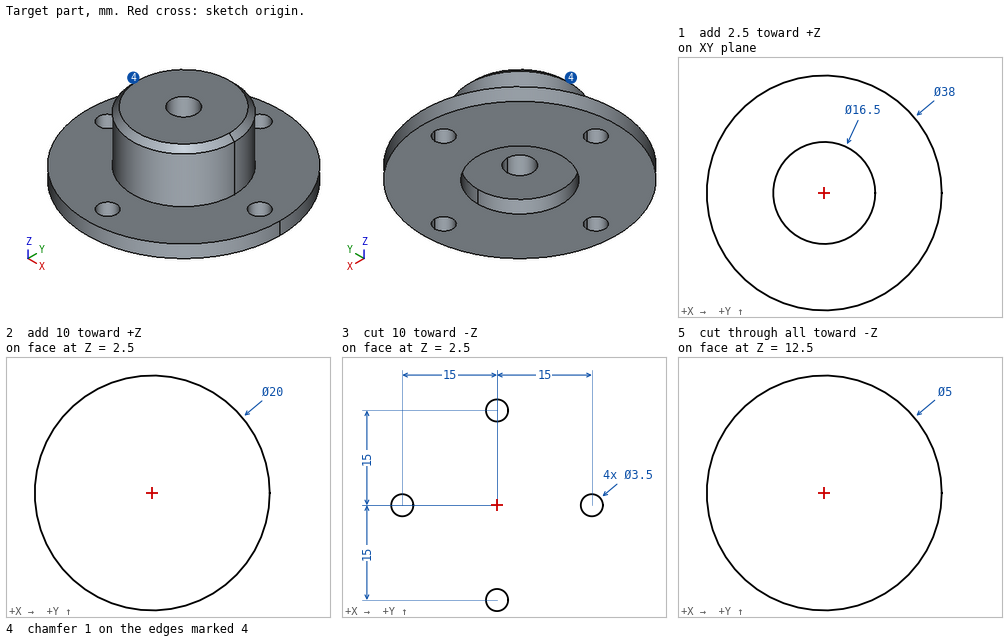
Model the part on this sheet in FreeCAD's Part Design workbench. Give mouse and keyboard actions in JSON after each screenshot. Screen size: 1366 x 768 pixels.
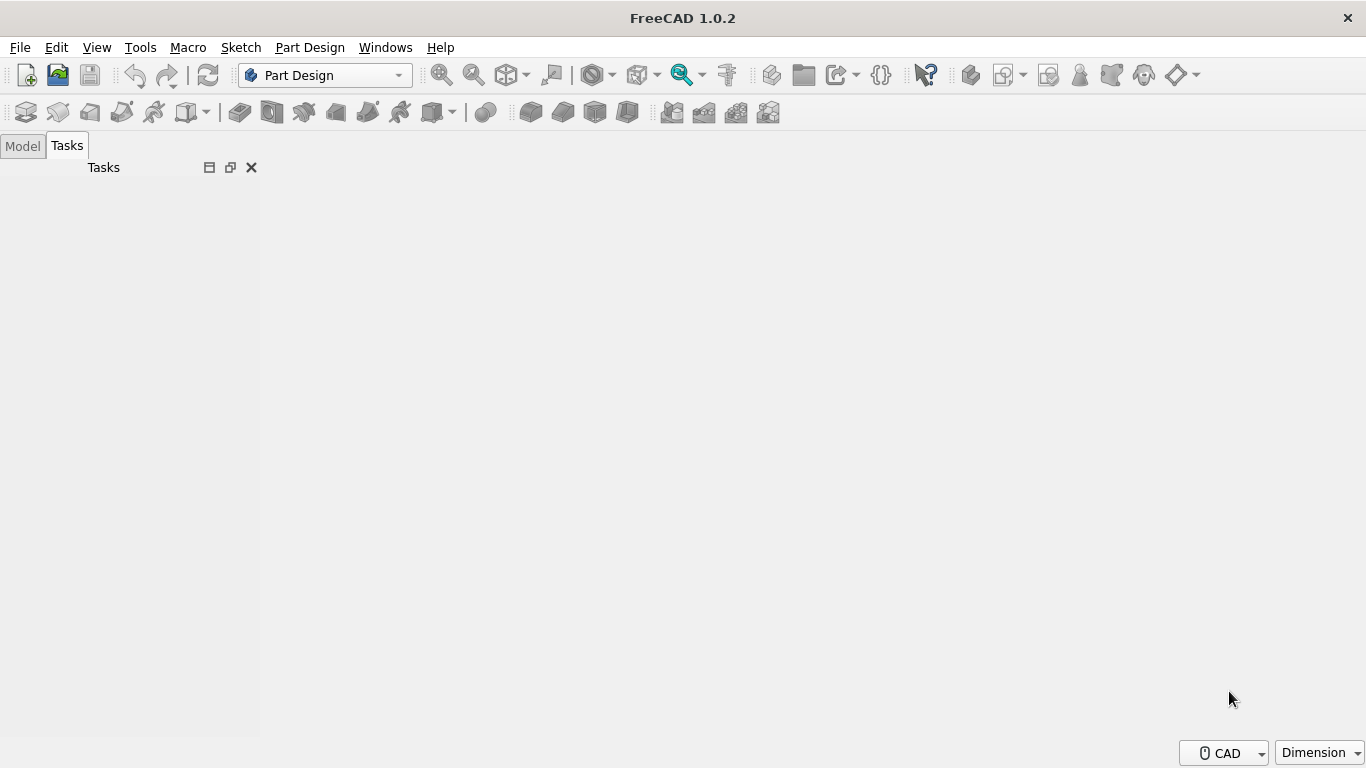
{"action": "key", "text": "ctrl+n"}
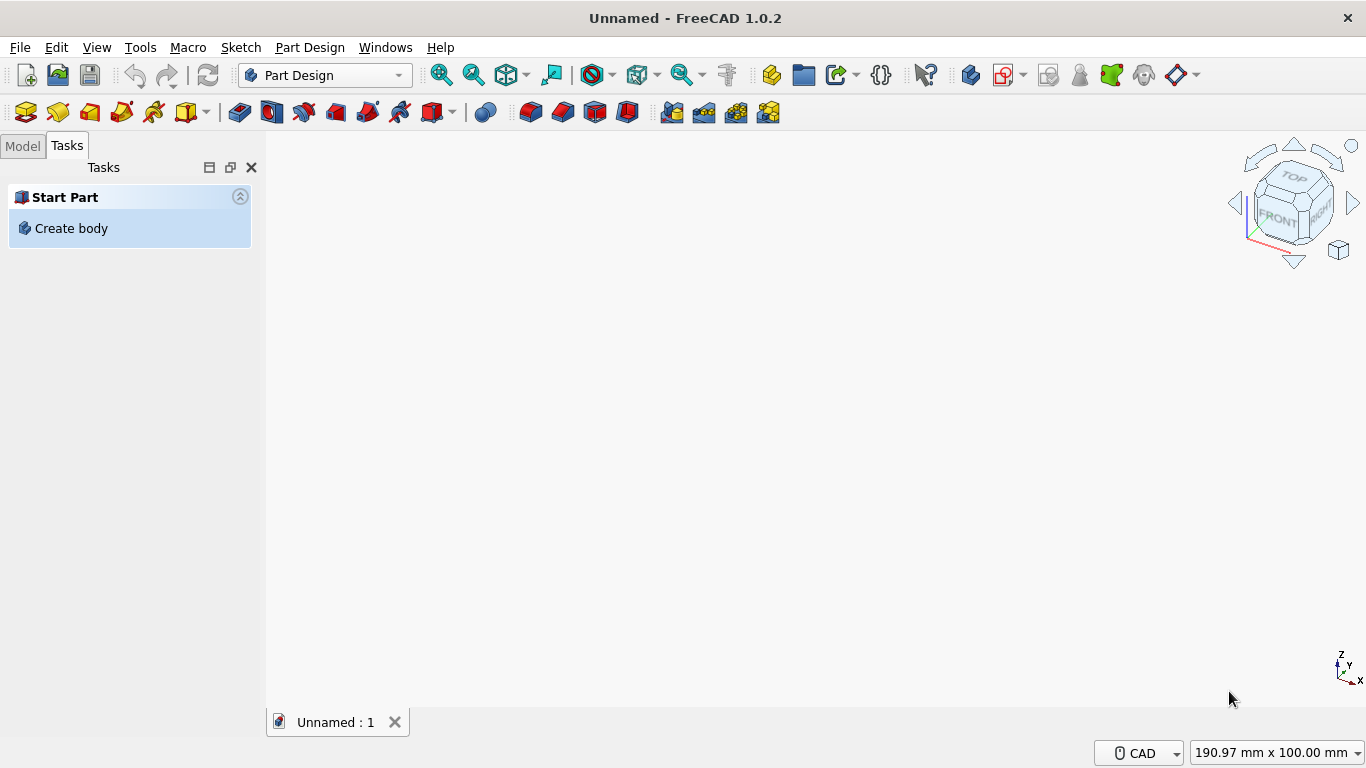
{"action": "left_click", "coordinate": [1004, 76]}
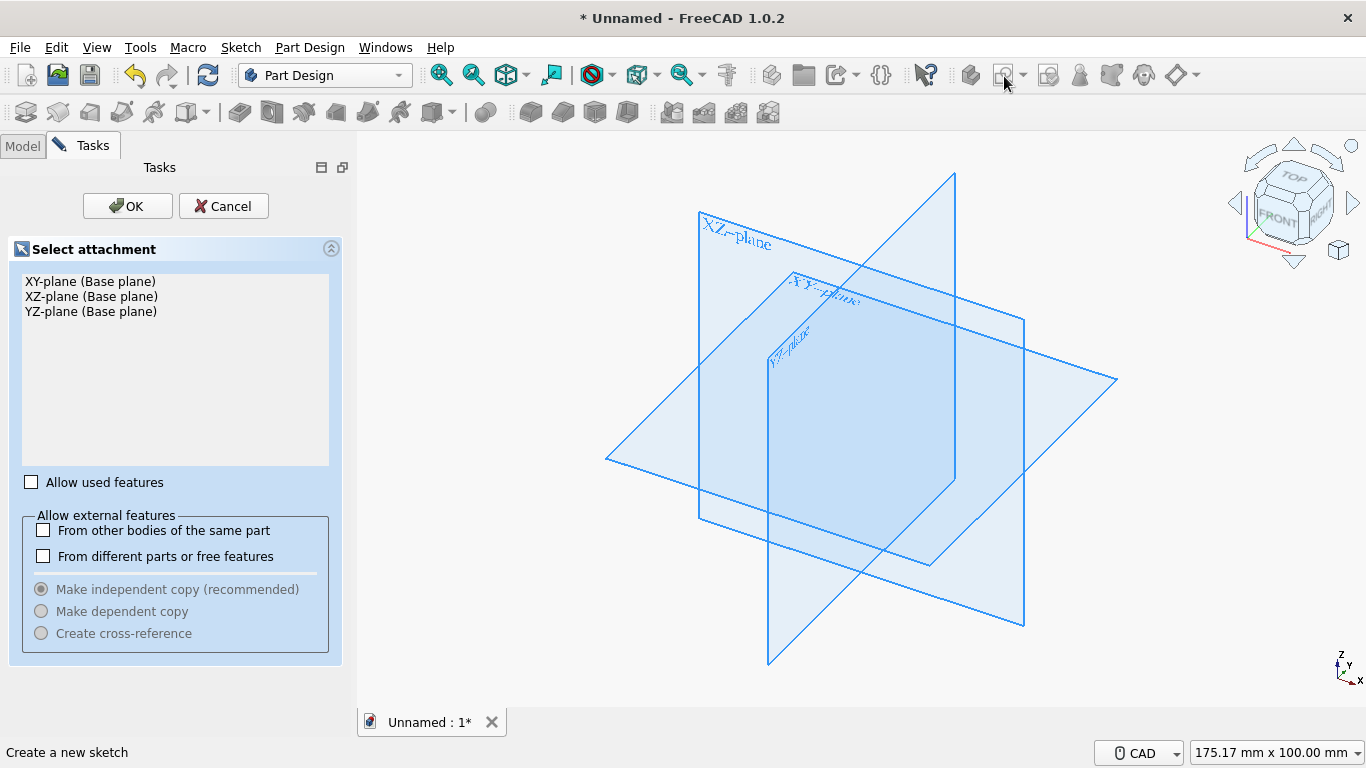
{"action": "left_click", "coordinate": [82, 282]}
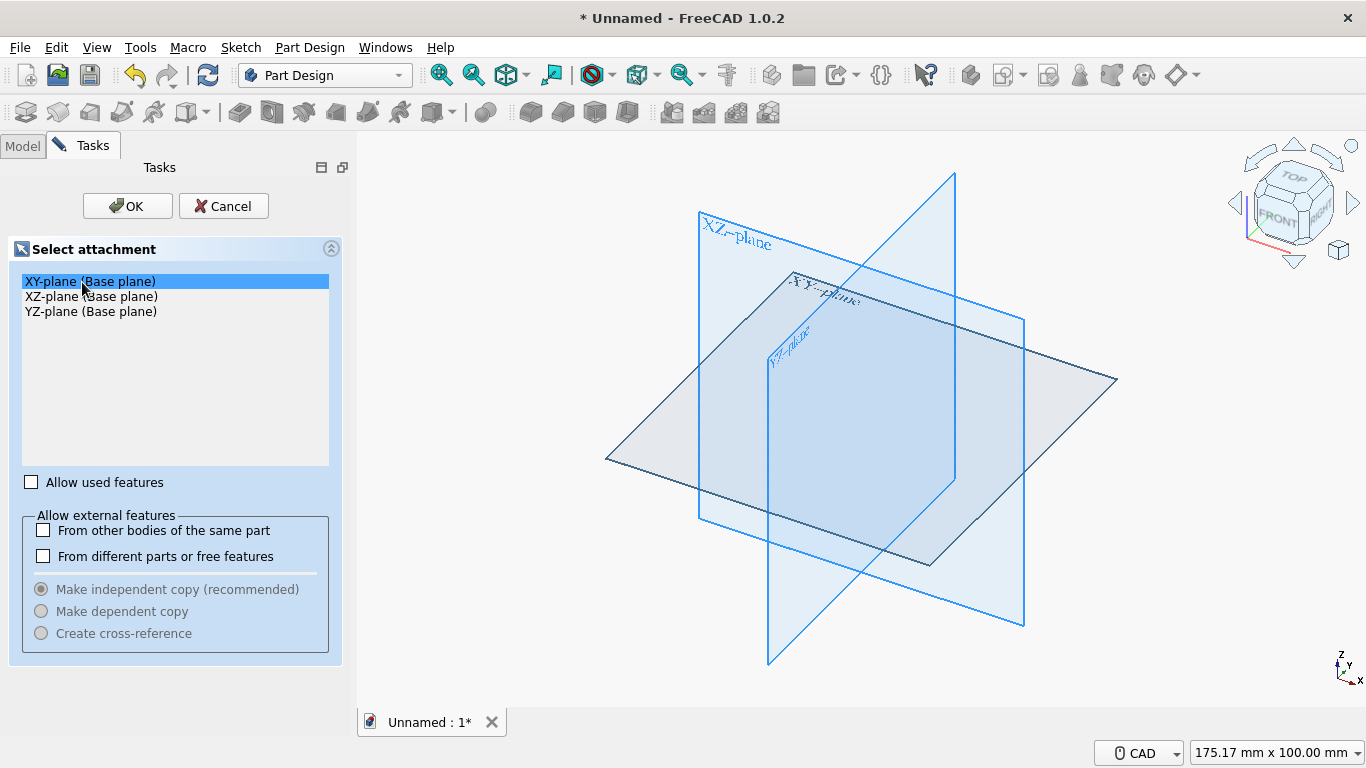
{"action": "left_click", "coordinate": [128, 206]}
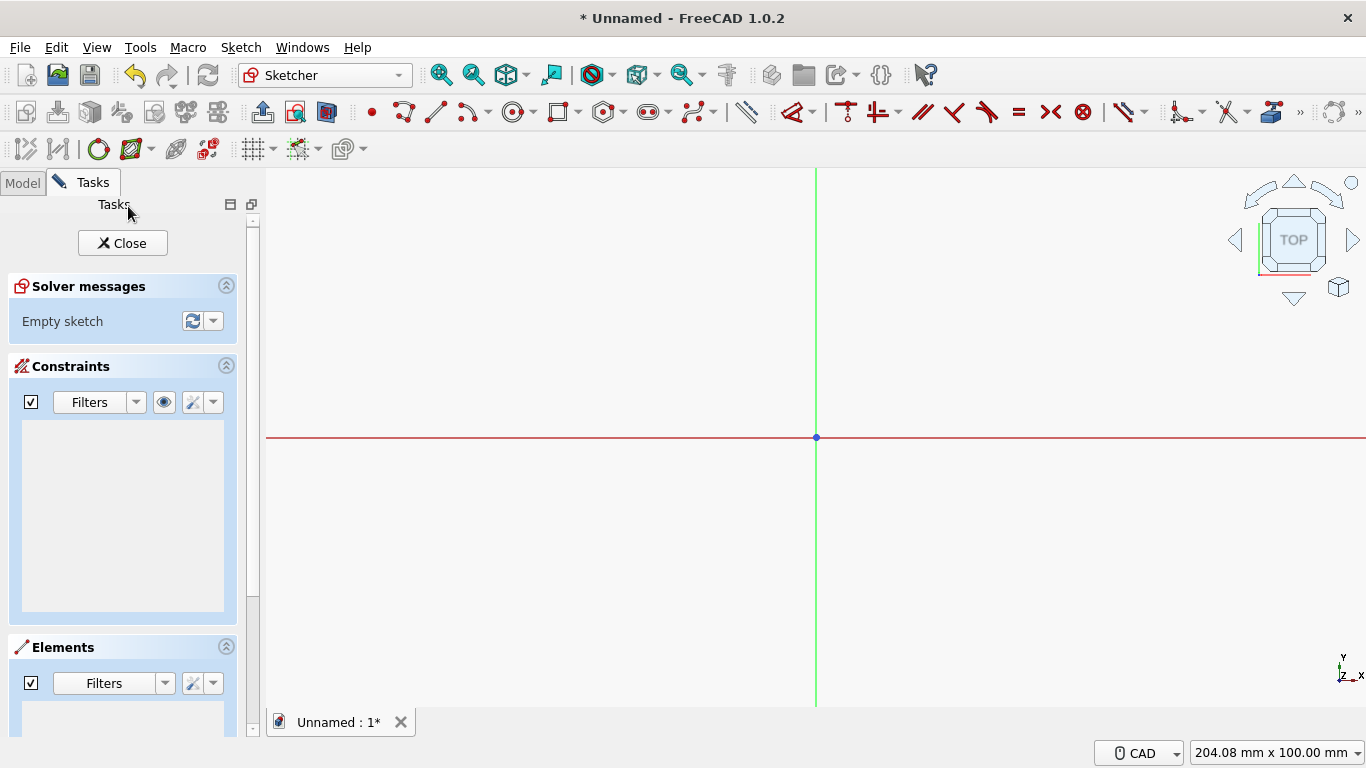
{"action": "scroll", "coordinate": [899, 438], "scroll_direction": "up", "scroll_amount": 3}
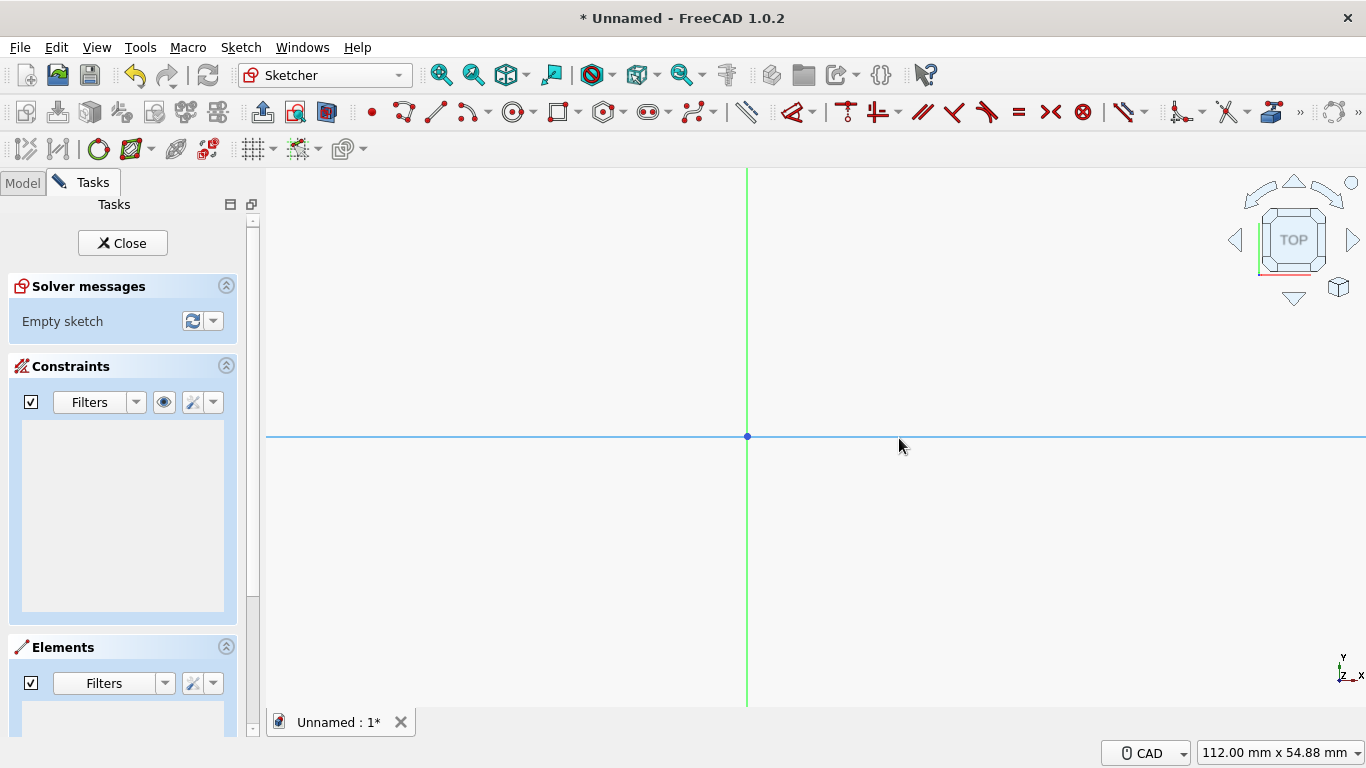
{"action": "key", "text": "g c"}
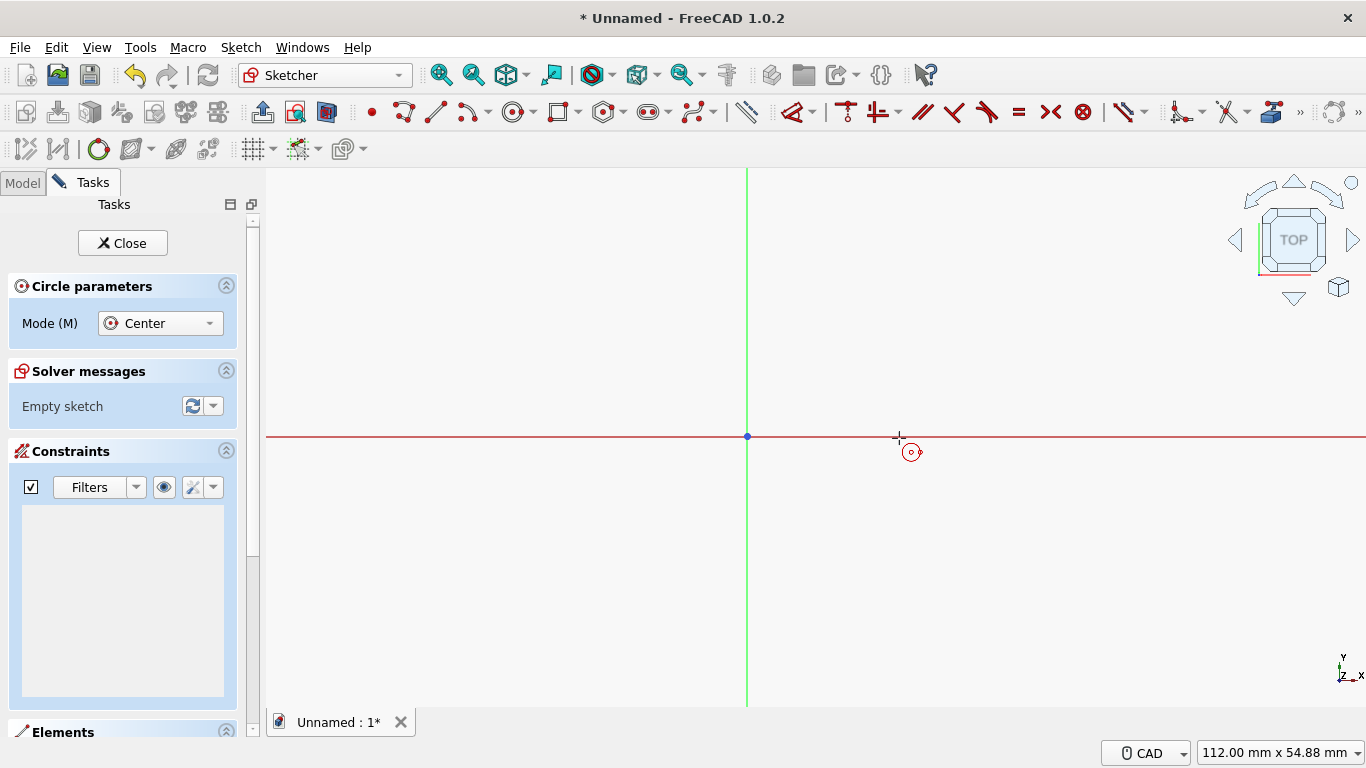
{"action": "left_click", "coordinate": [747, 437]}
{"action": "mouse_move", "coordinate": [879, 305]}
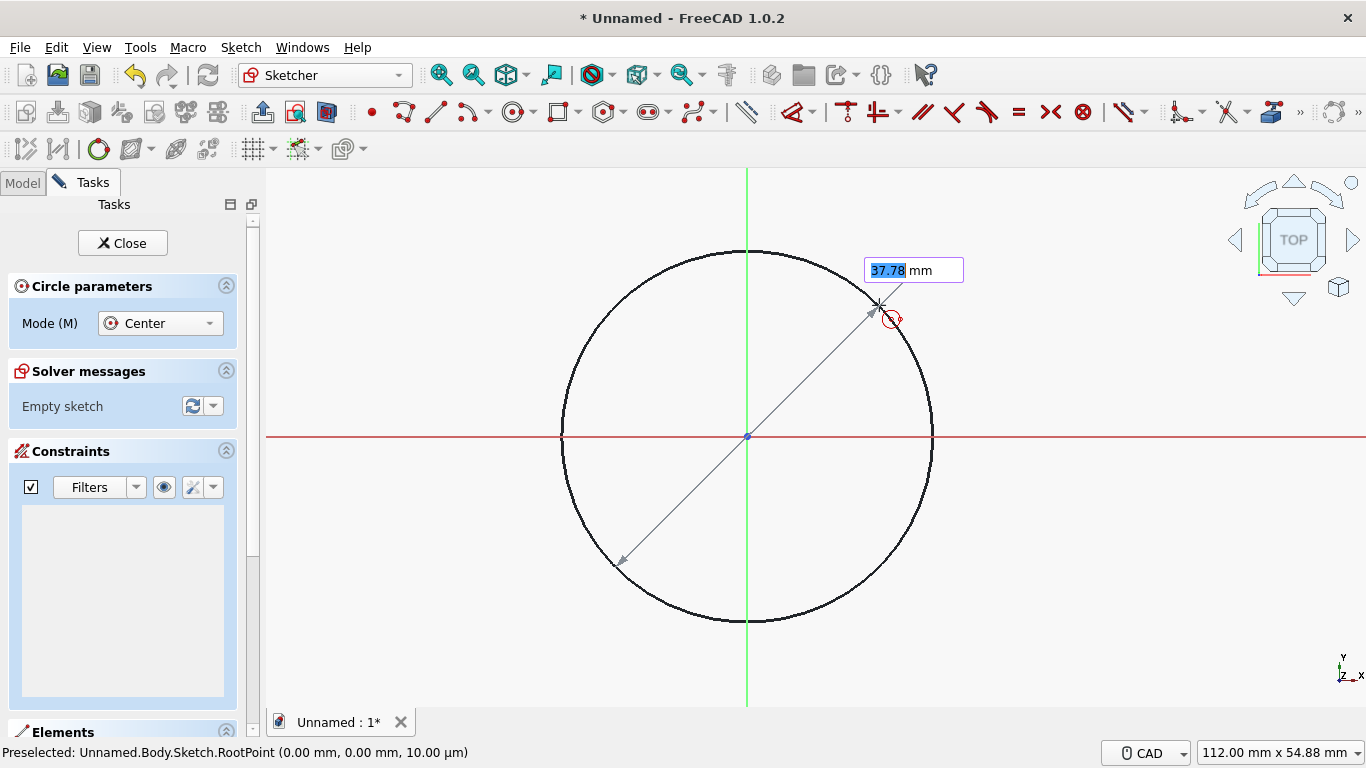
{"action": "type", "text": "38"}
{"action": "key", "text": "Return"}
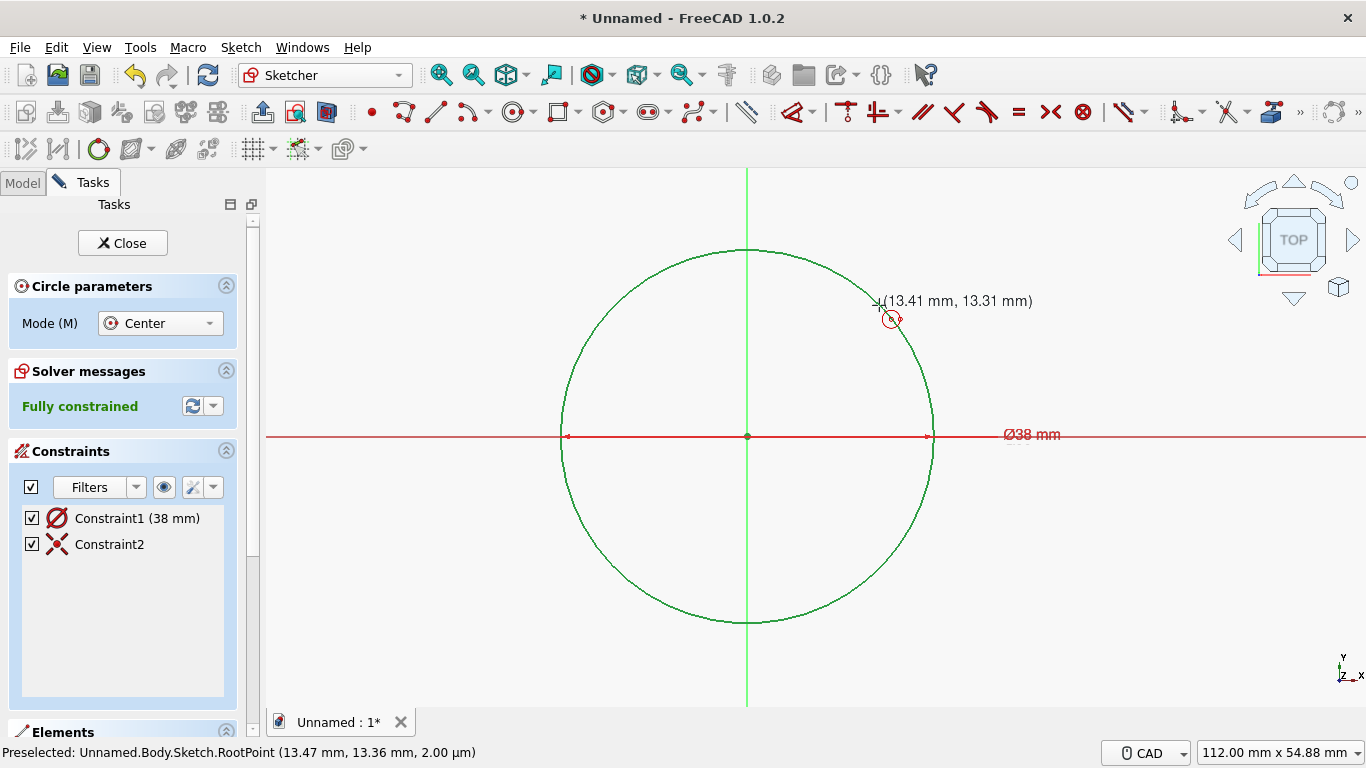
{"action": "left_click", "coordinate": [747, 437]}
{"action": "mouse_move", "coordinate": [805, 379]}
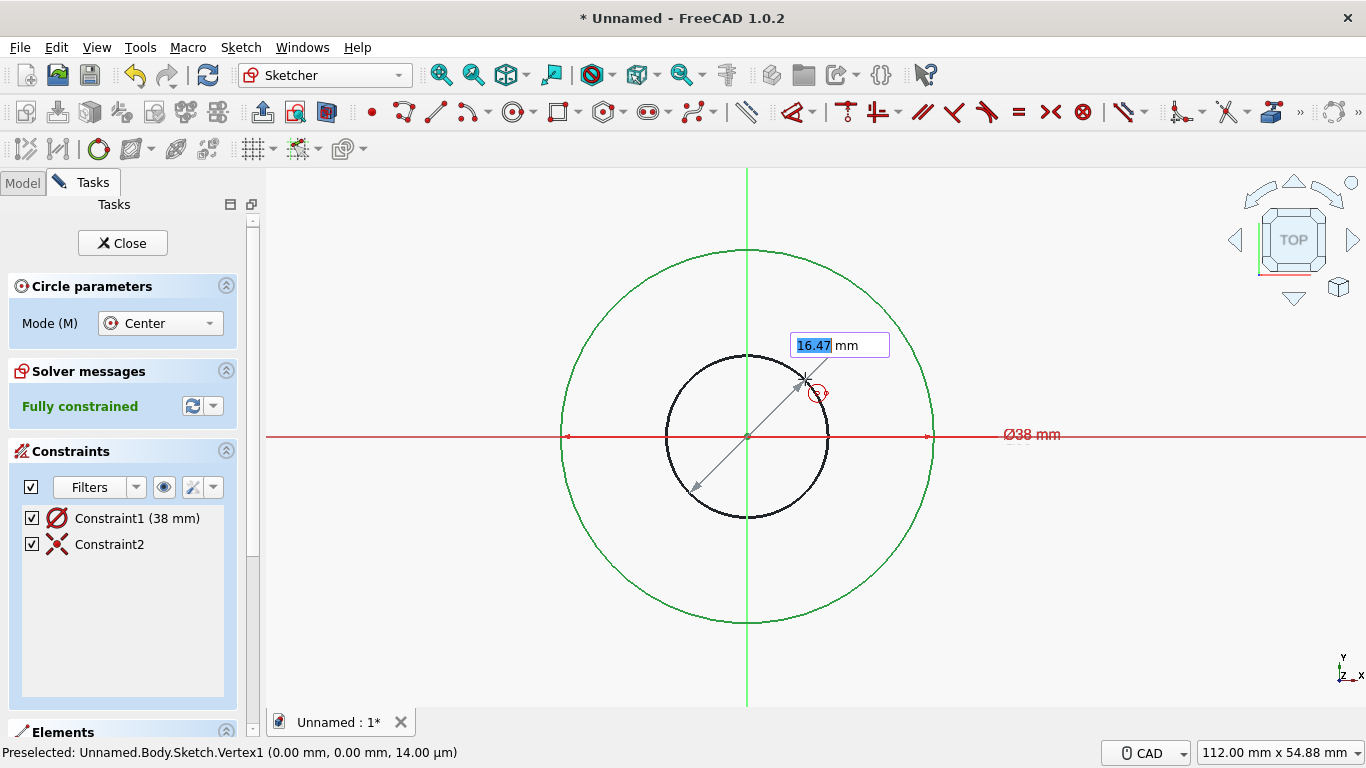
{"action": "type", "text": "16.5"}
{"action": "key", "text": "Return"}
{"action": "key", "text": "Escape"}